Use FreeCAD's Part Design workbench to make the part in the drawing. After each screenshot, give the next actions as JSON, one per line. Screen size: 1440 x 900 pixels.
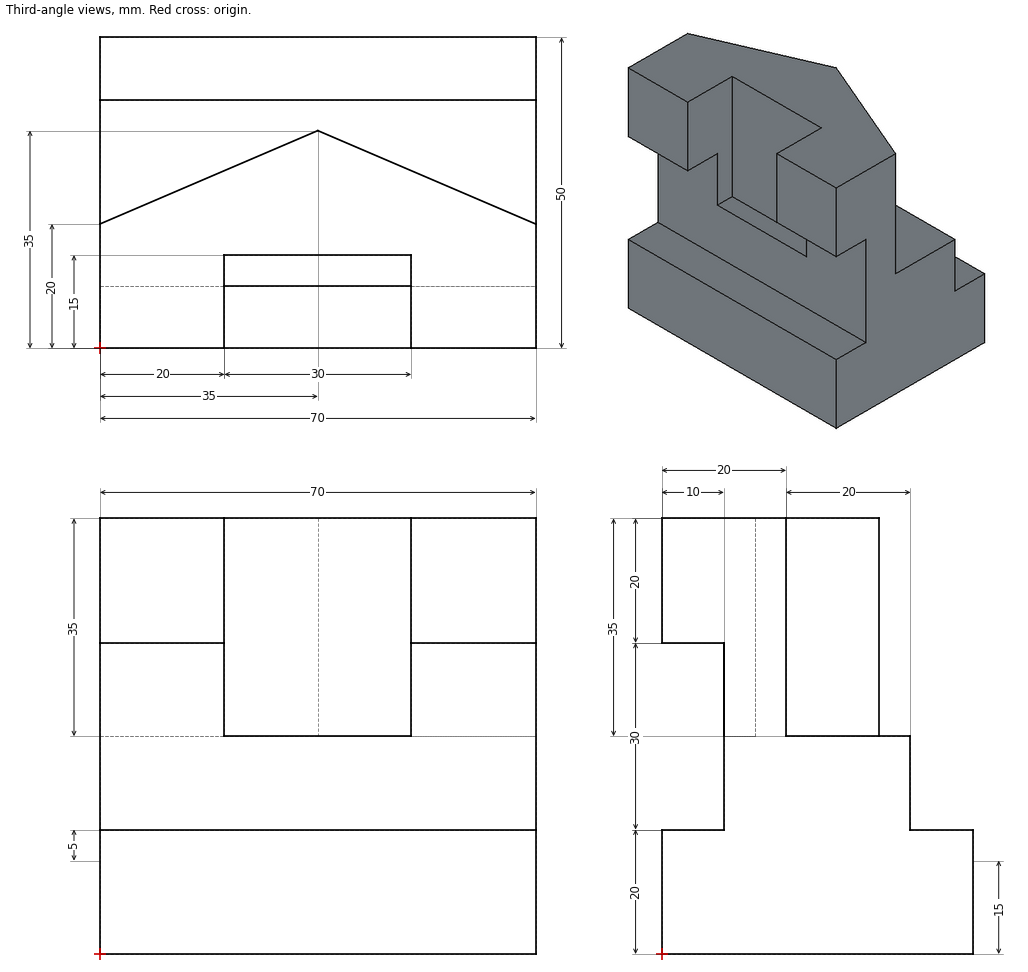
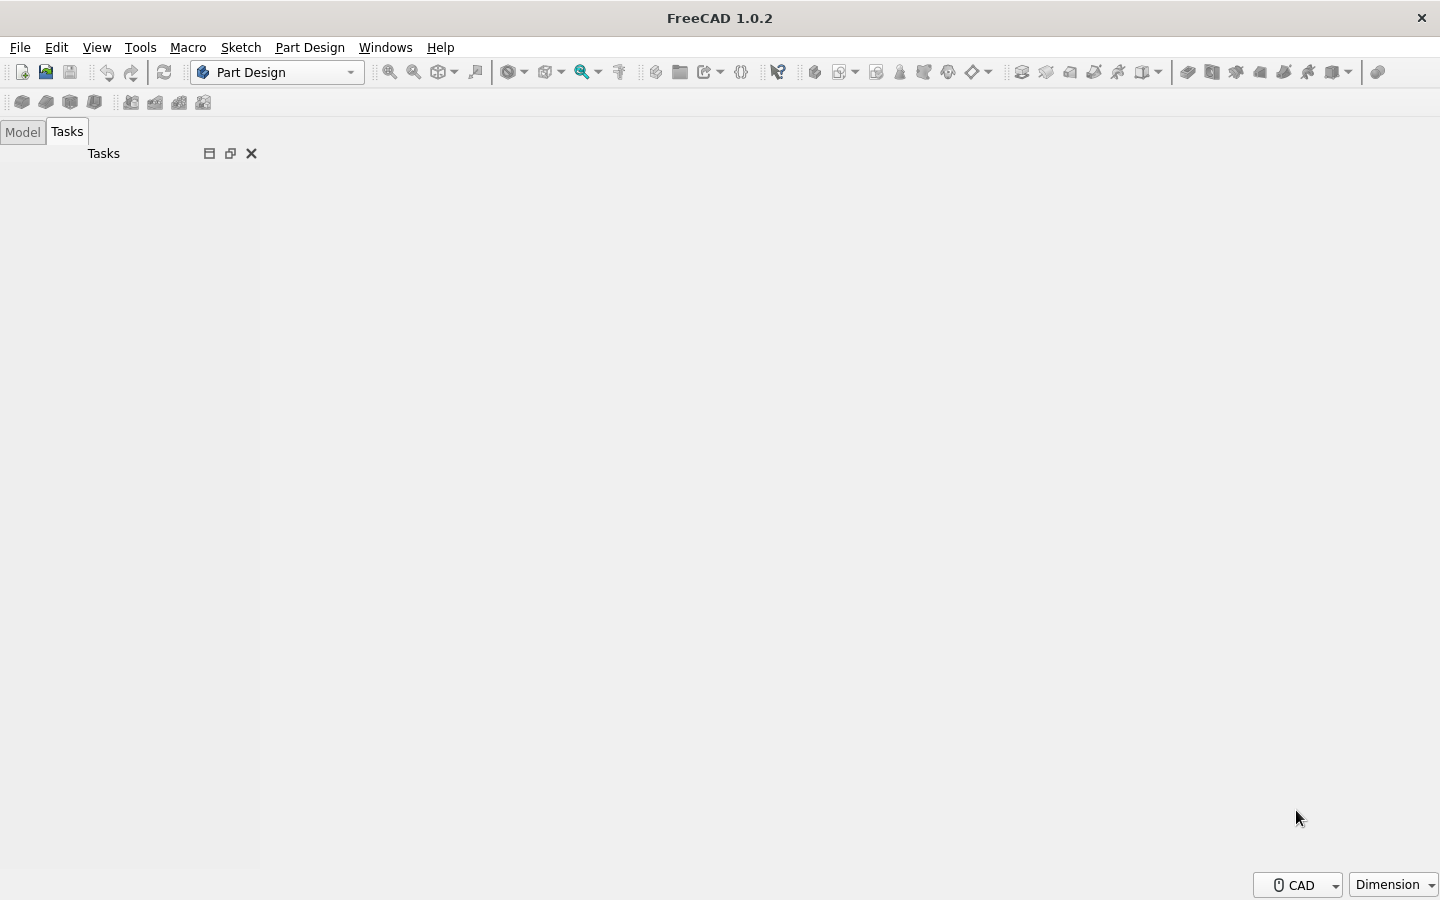
{"action": "left_click", "coordinate": [22, 72]}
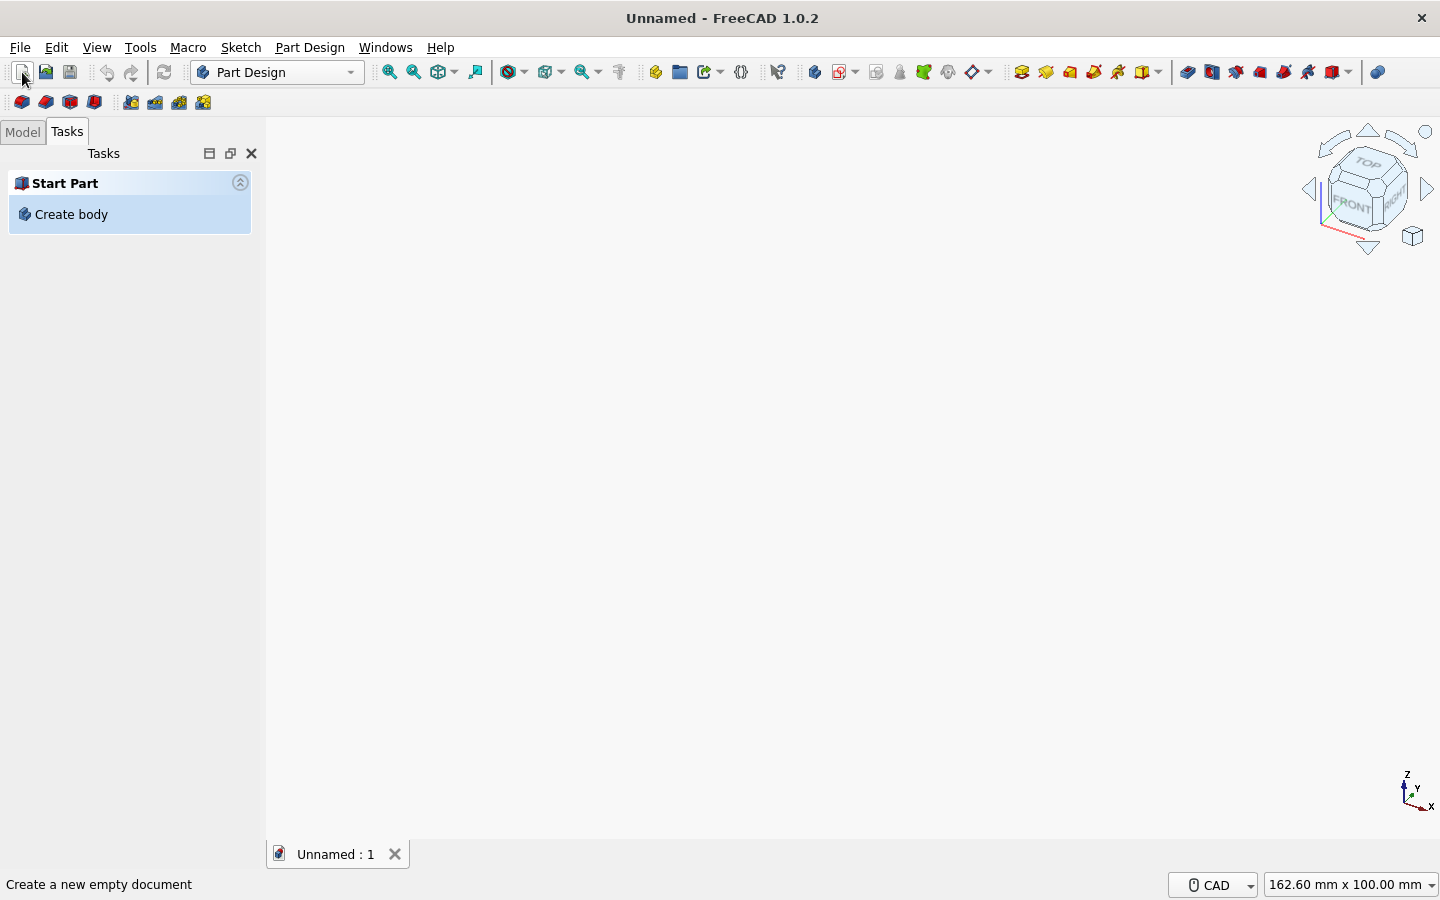
{"action": "left_click", "coordinate": [840, 72]}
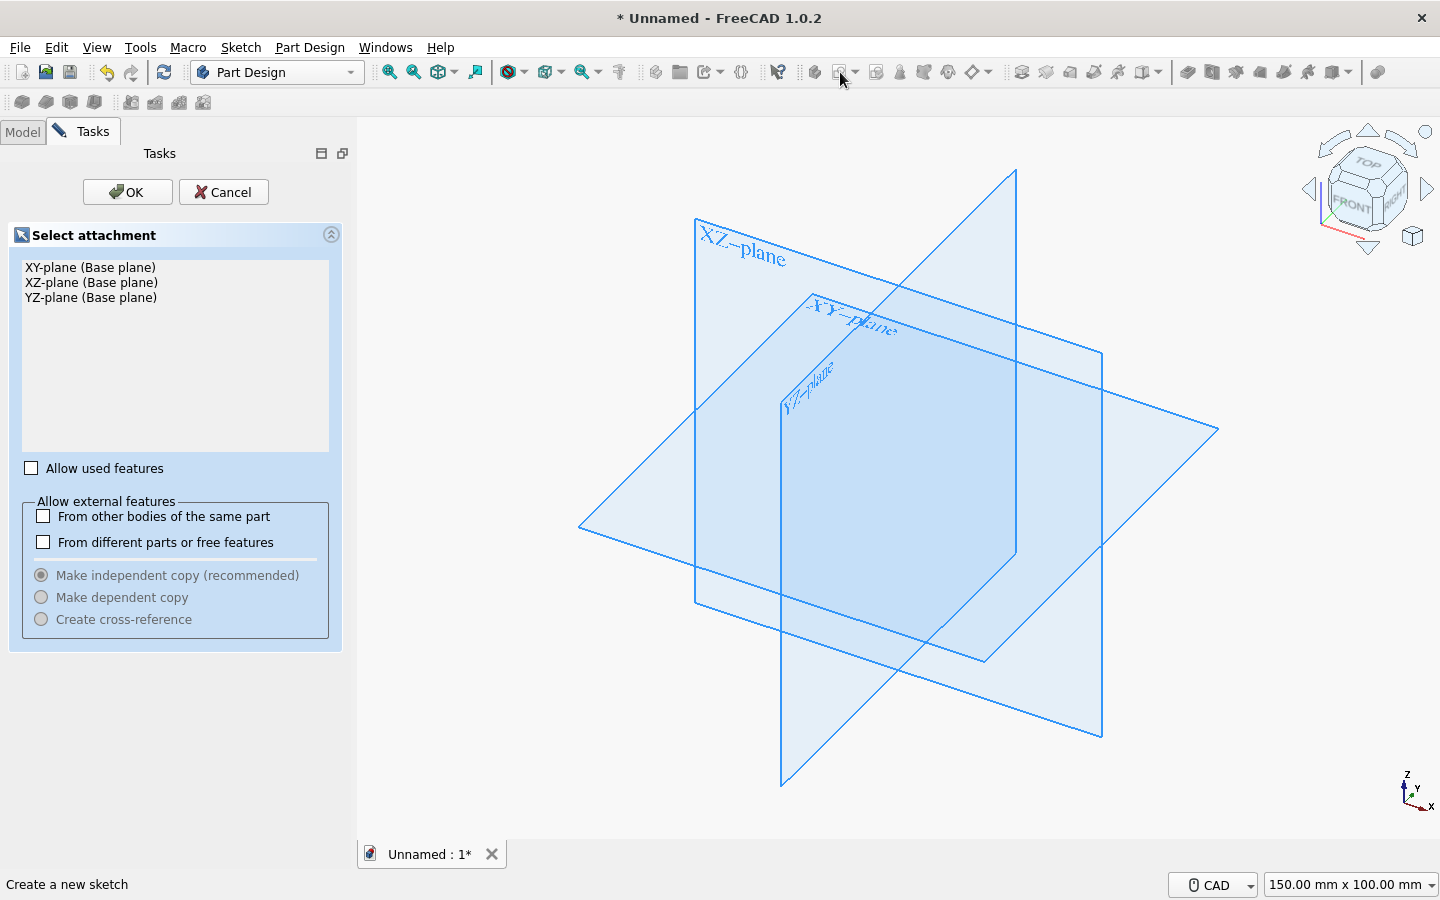
{"action": "left_click", "coordinate": [82, 268]}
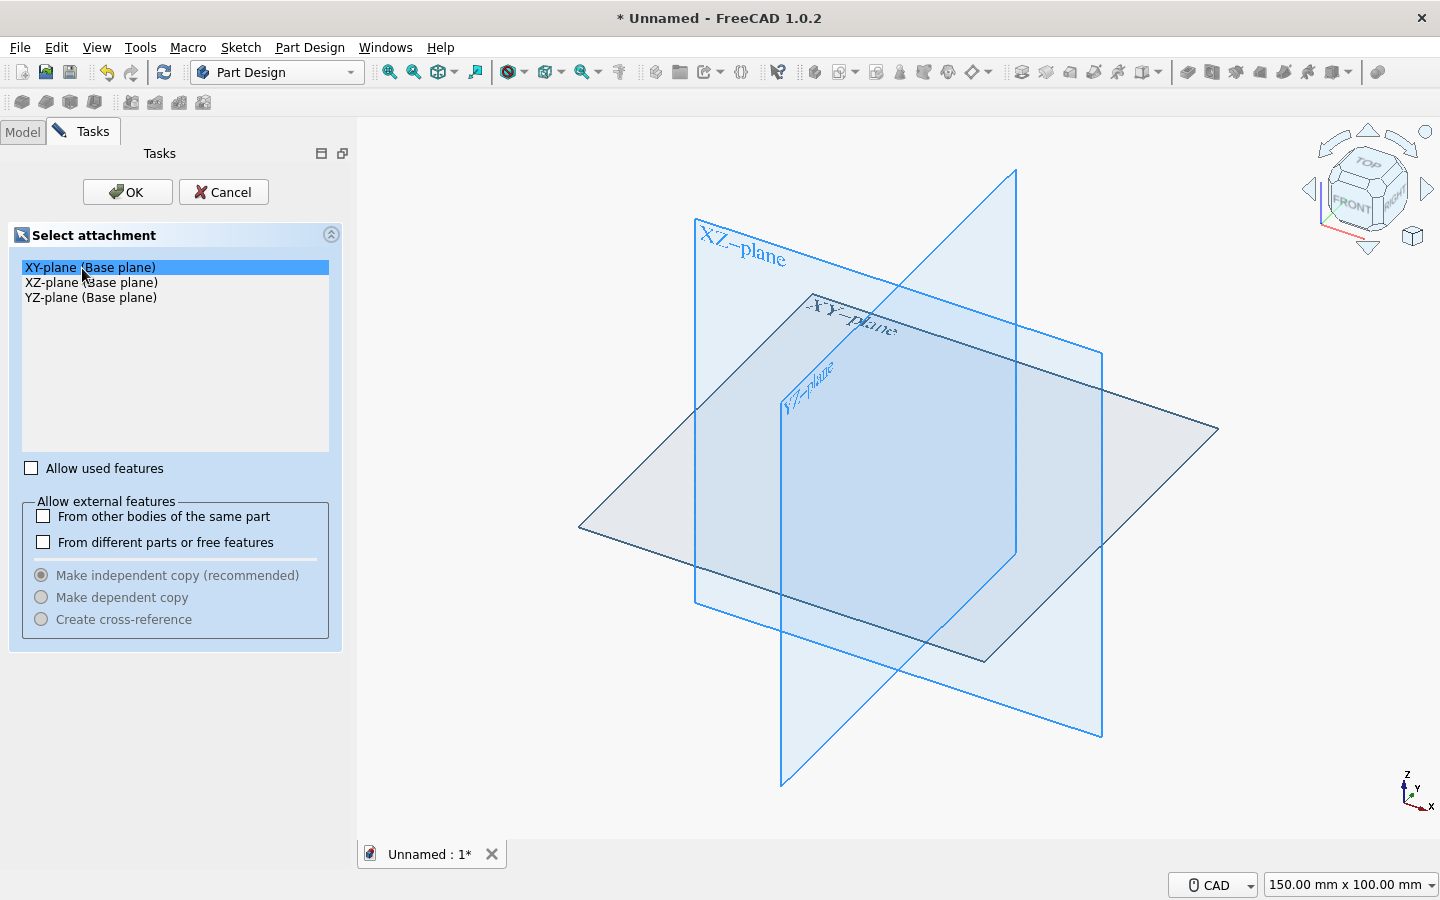
{"action": "left_click", "coordinate": [128, 192]}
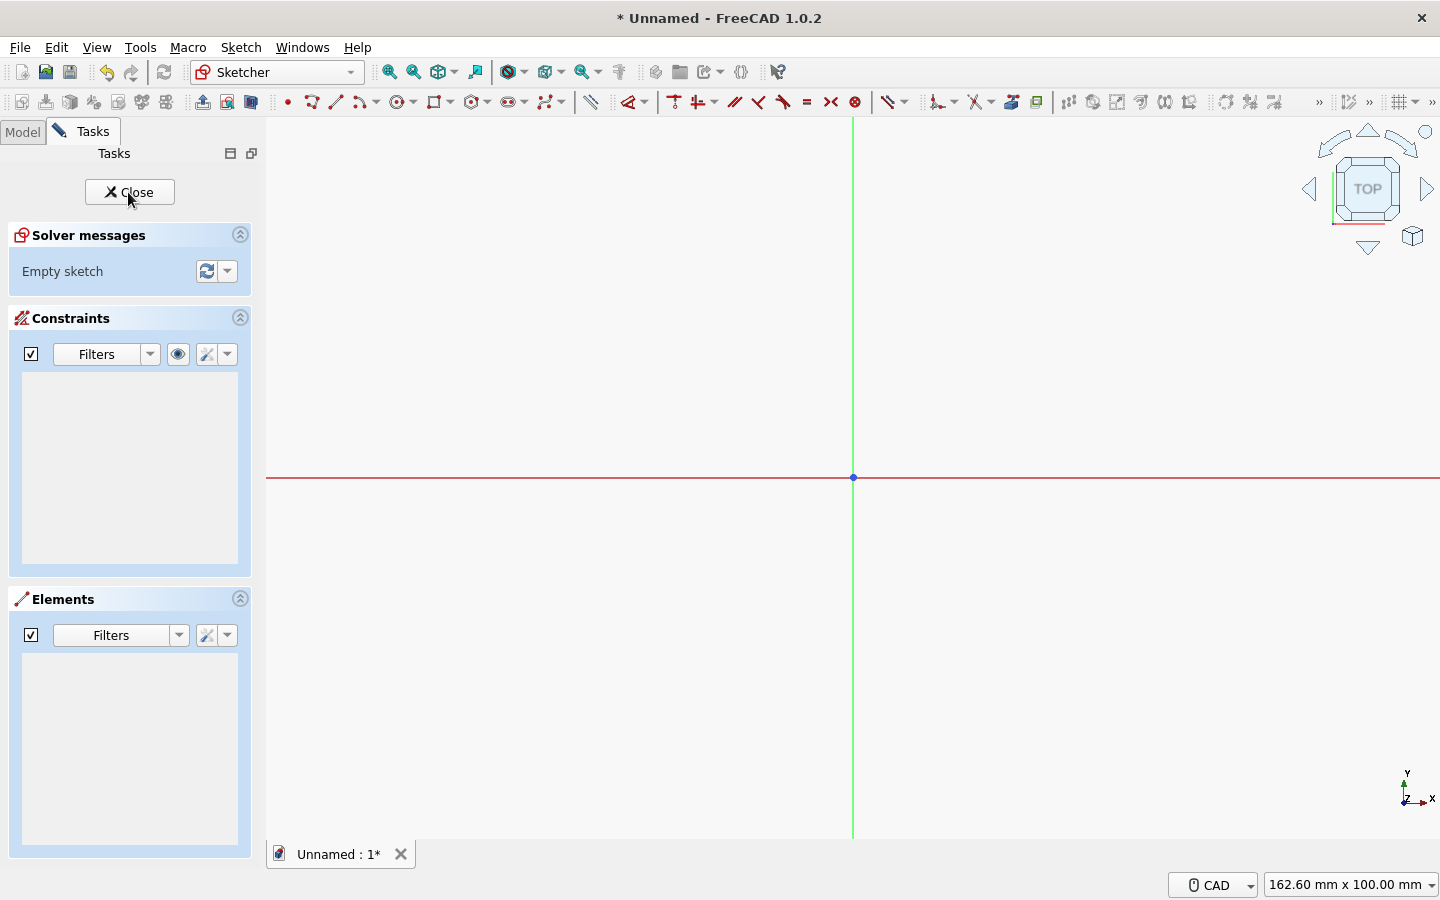
{"action": "scroll", "coordinate": [294, 811], "scroll_direction": "down", "scroll_amount": 1}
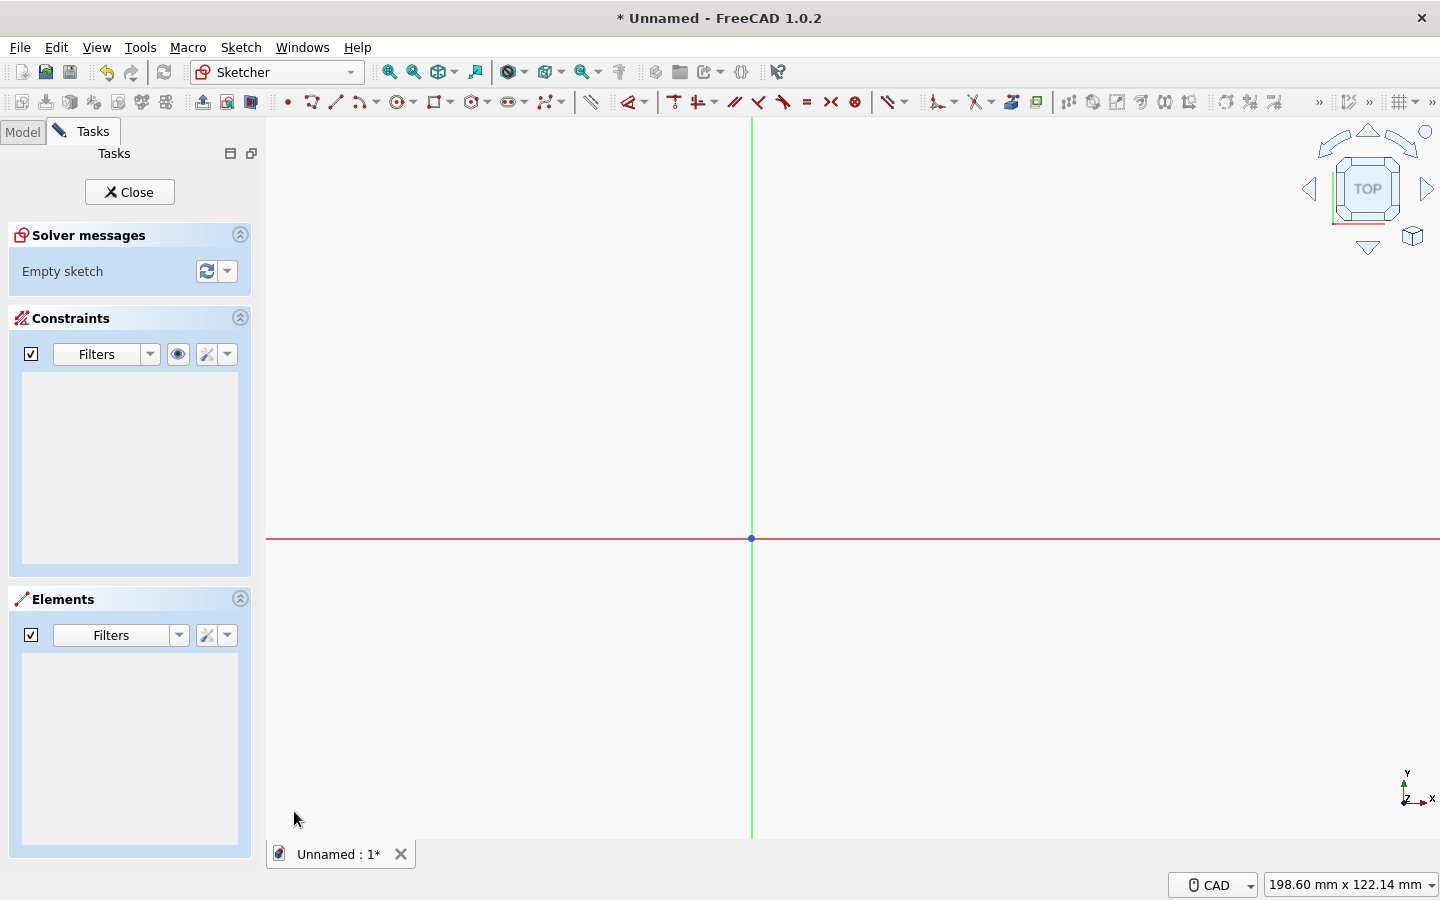
{"action": "scroll", "coordinate": [1275, 213], "scroll_direction": "up", "scroll_amount": 2}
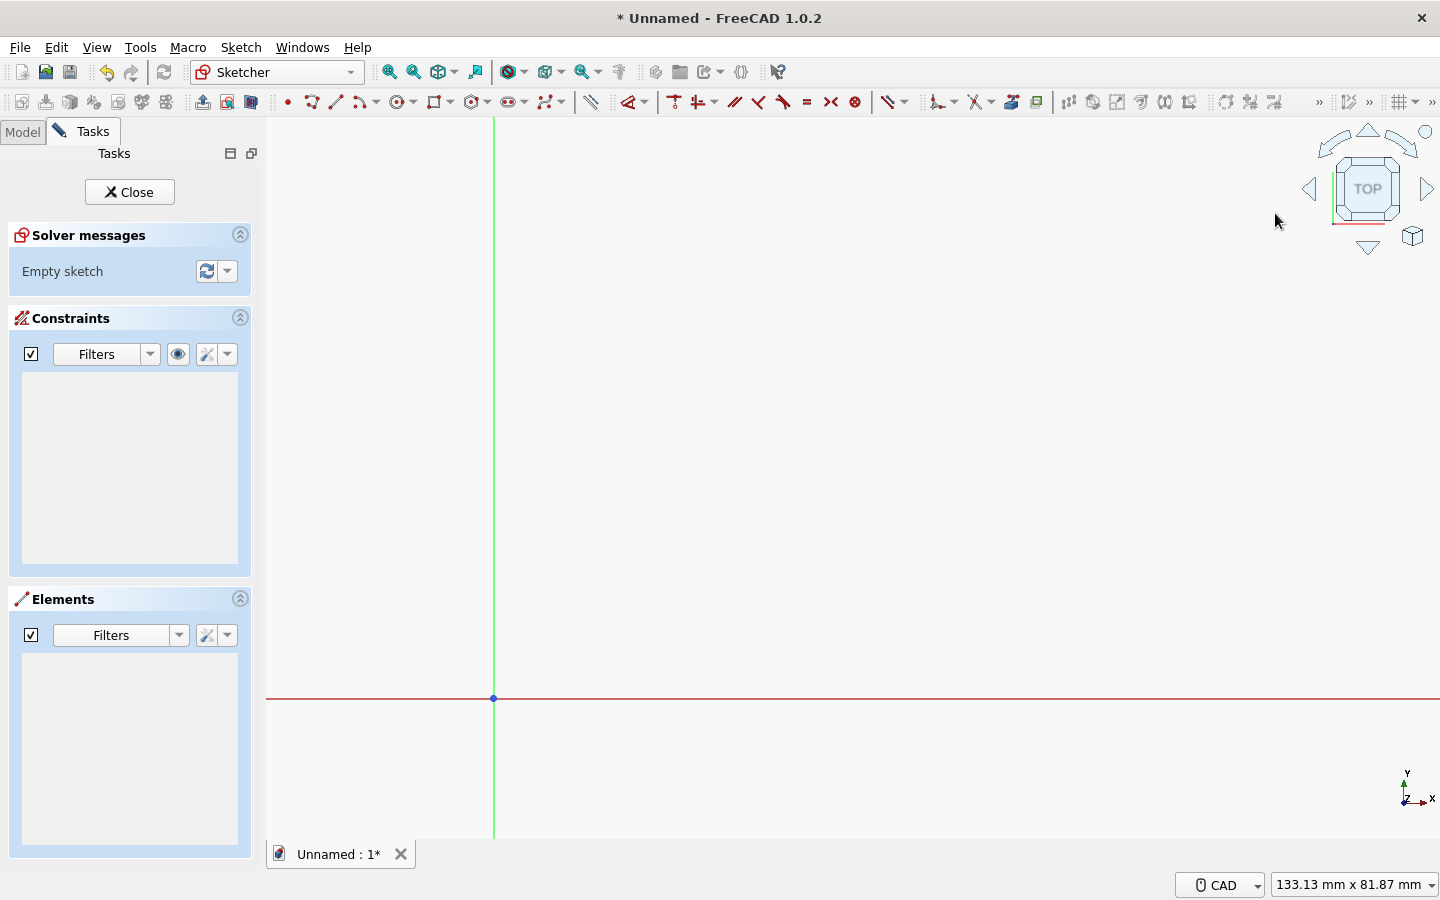
{"action": "left_click", "coordinate": [434, 102]}